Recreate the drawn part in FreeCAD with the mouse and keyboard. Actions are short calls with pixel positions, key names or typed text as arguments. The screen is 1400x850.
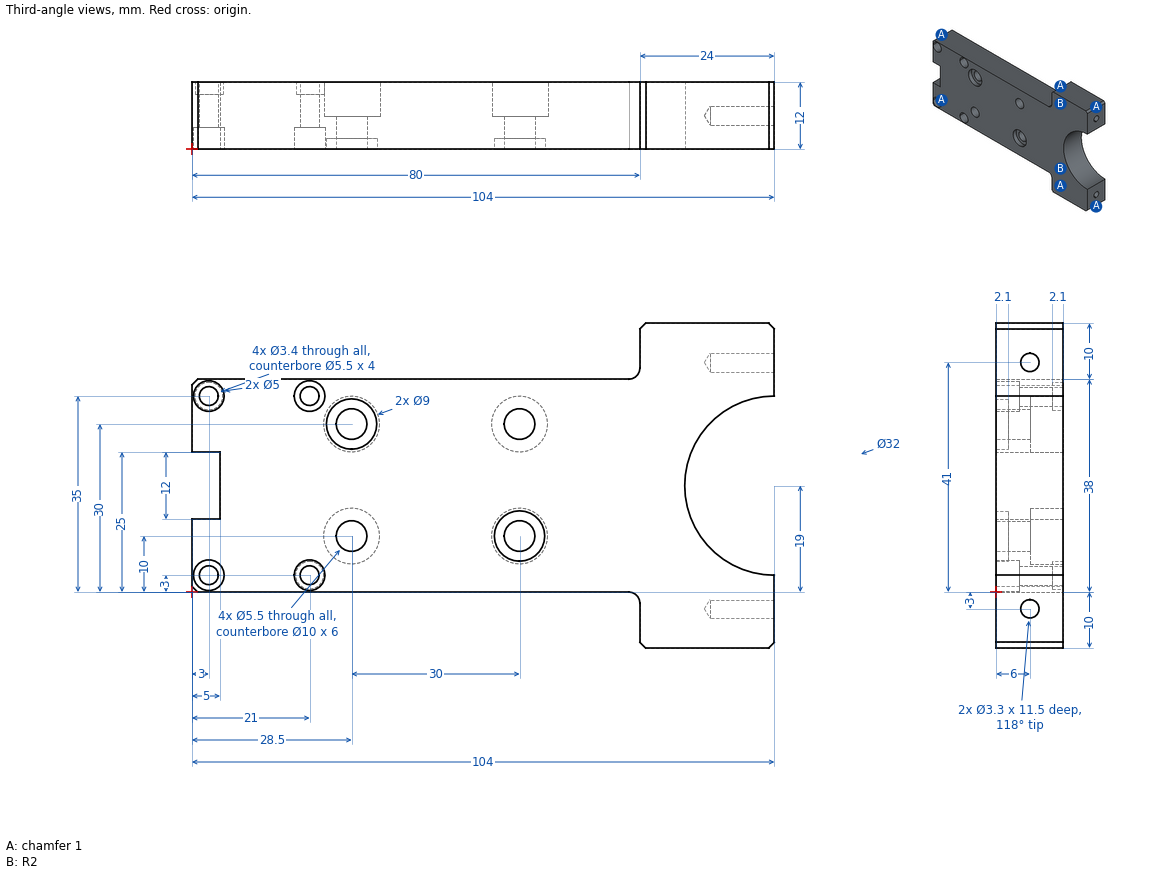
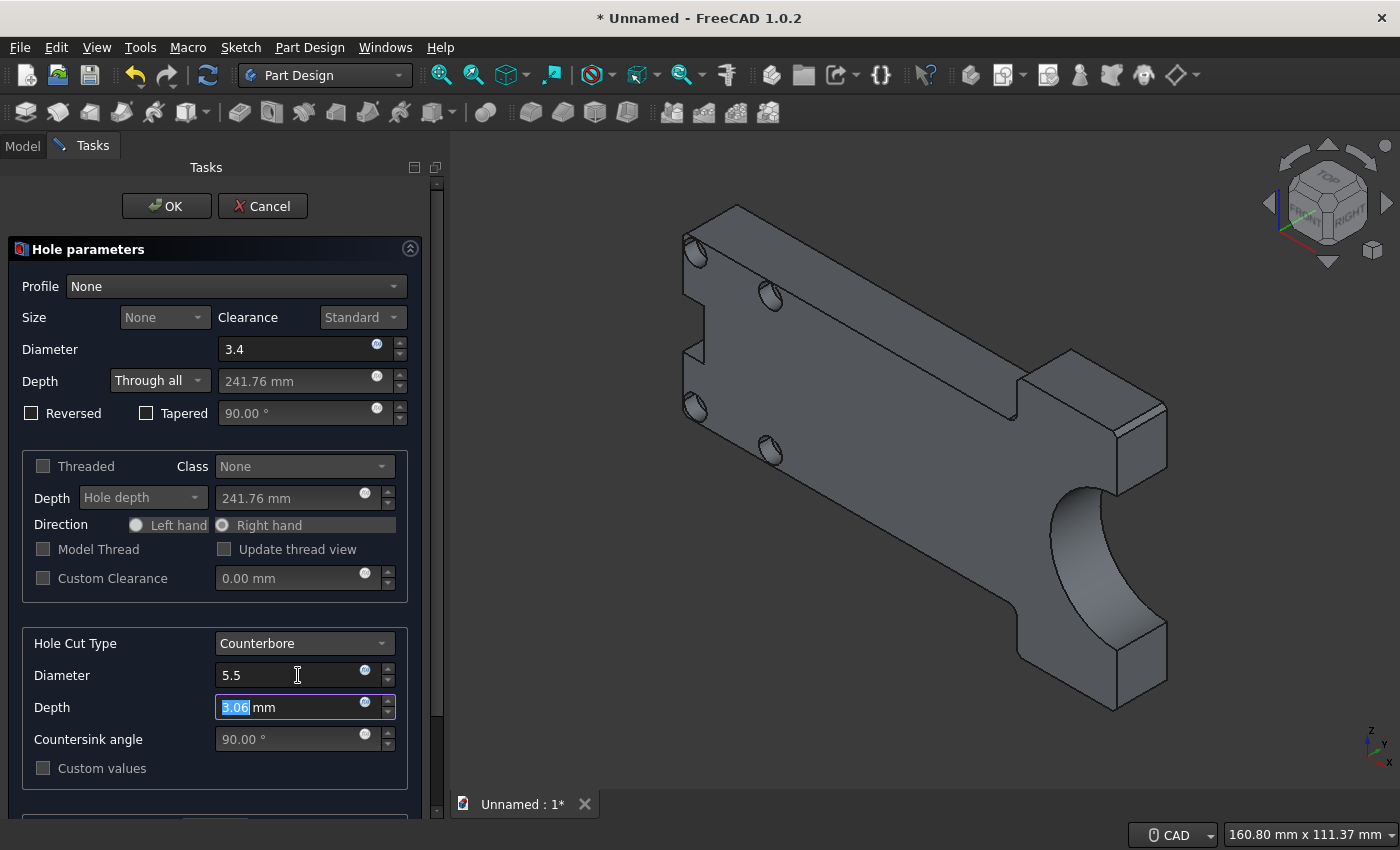
text(4)
key(Tab)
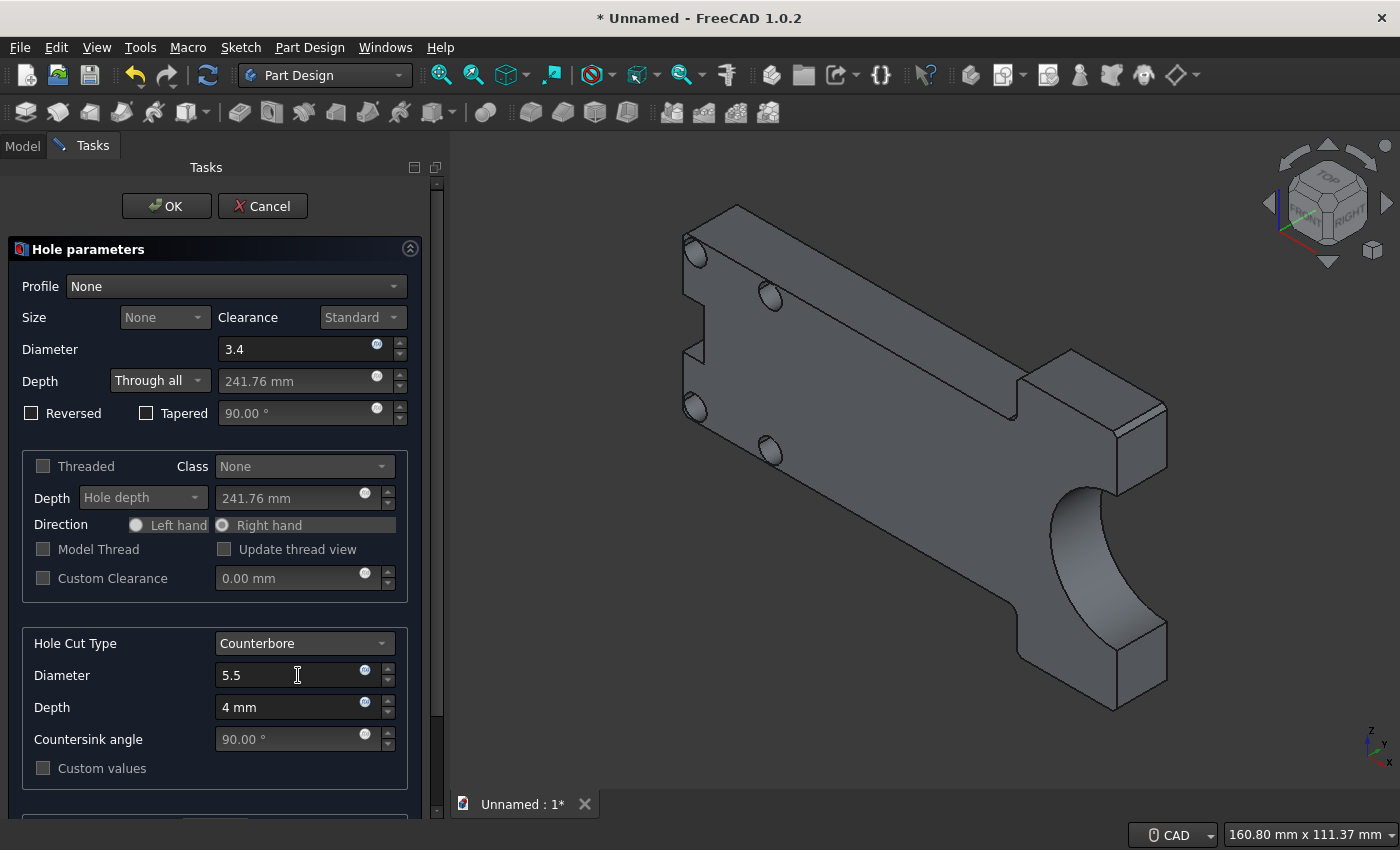
click(167, 206)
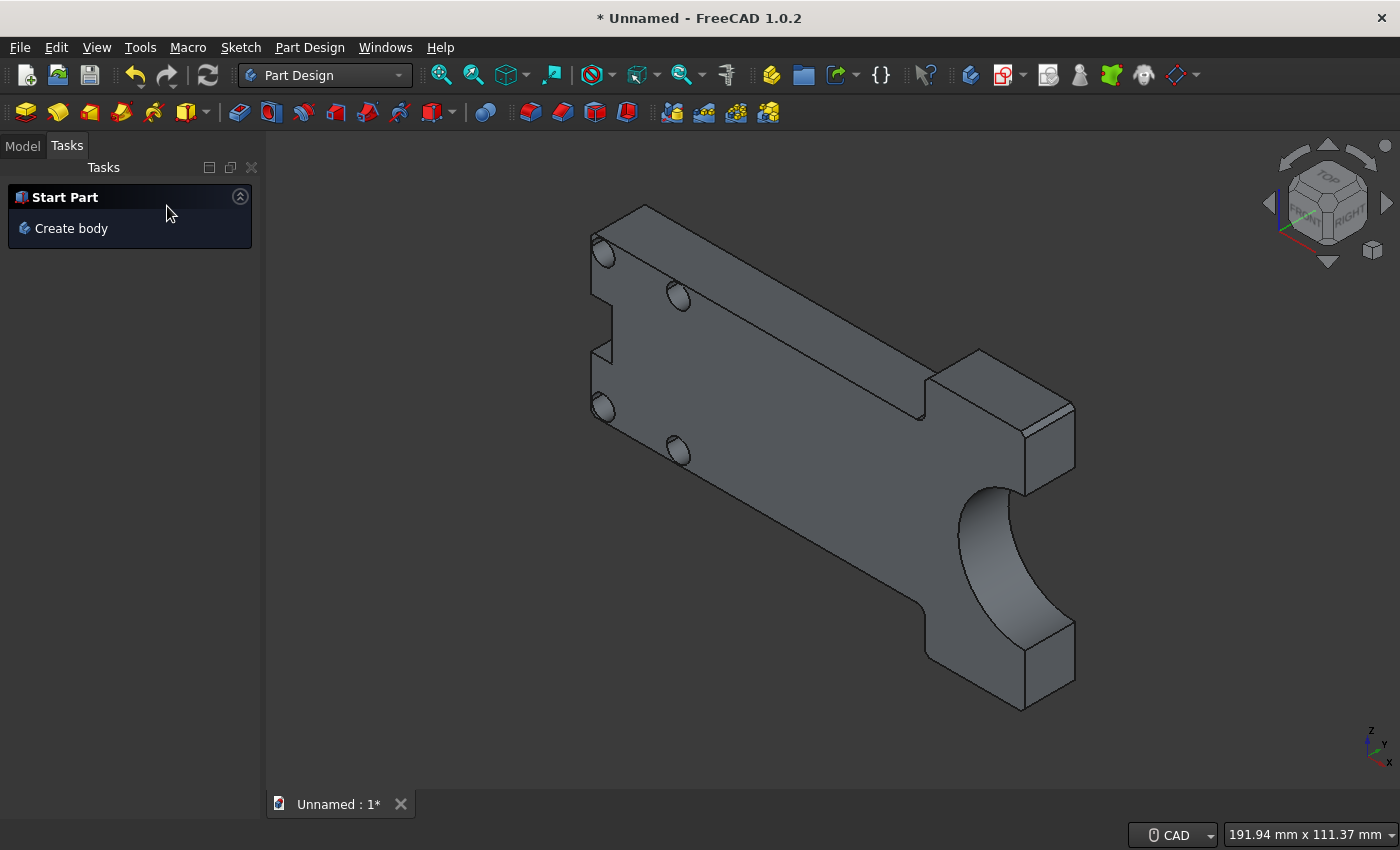
key(4)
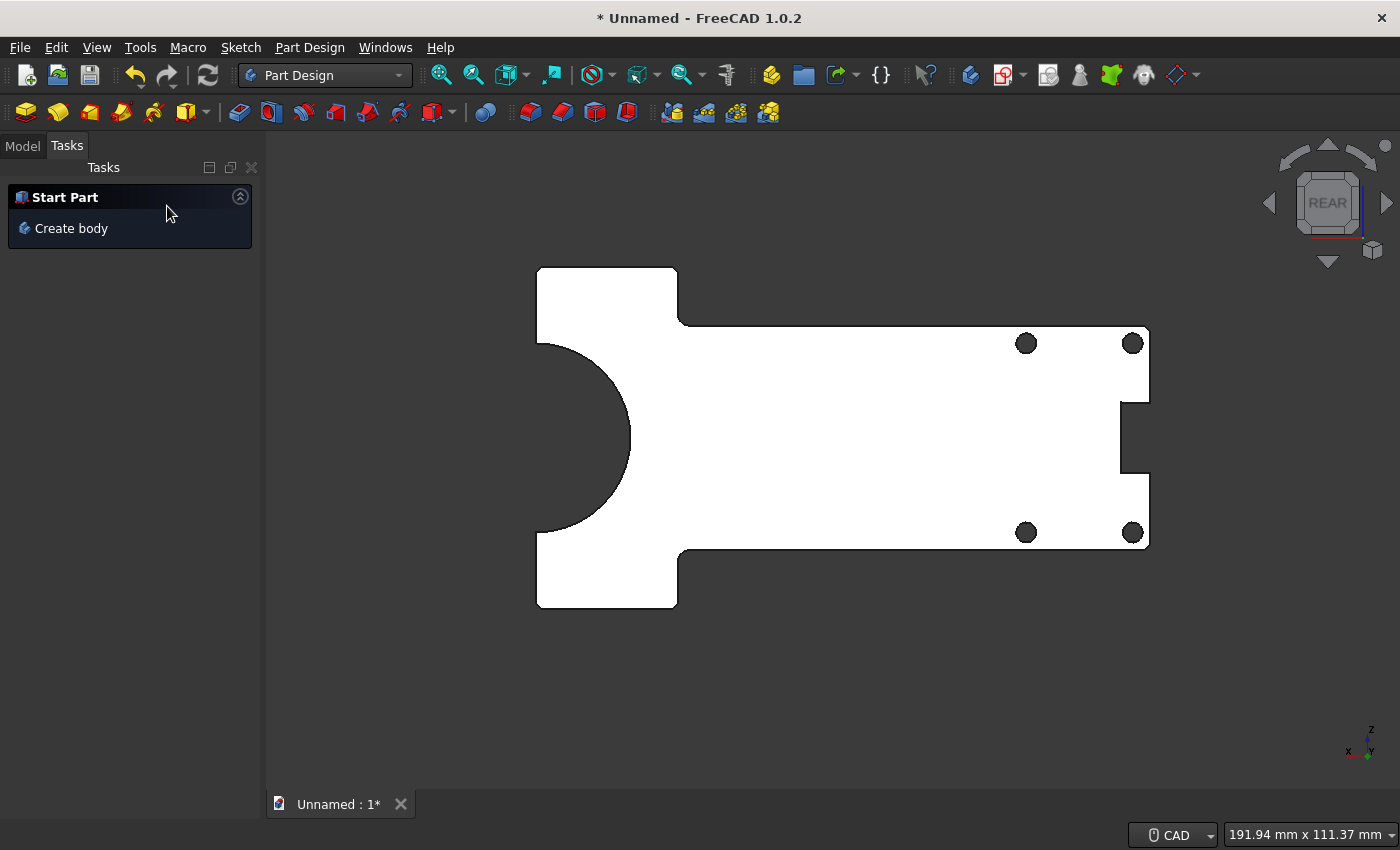
click(755, 437)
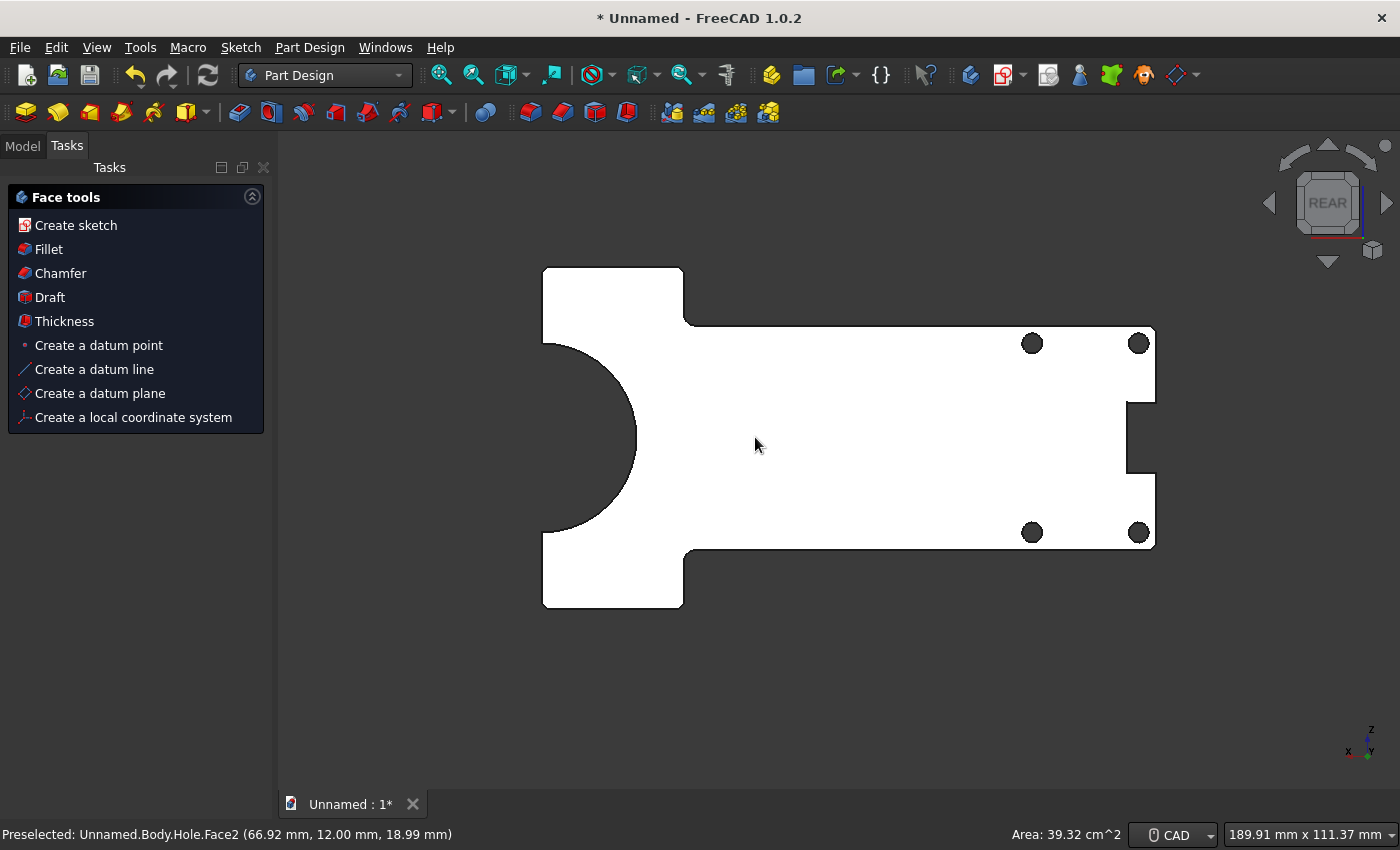
click(1004, 76)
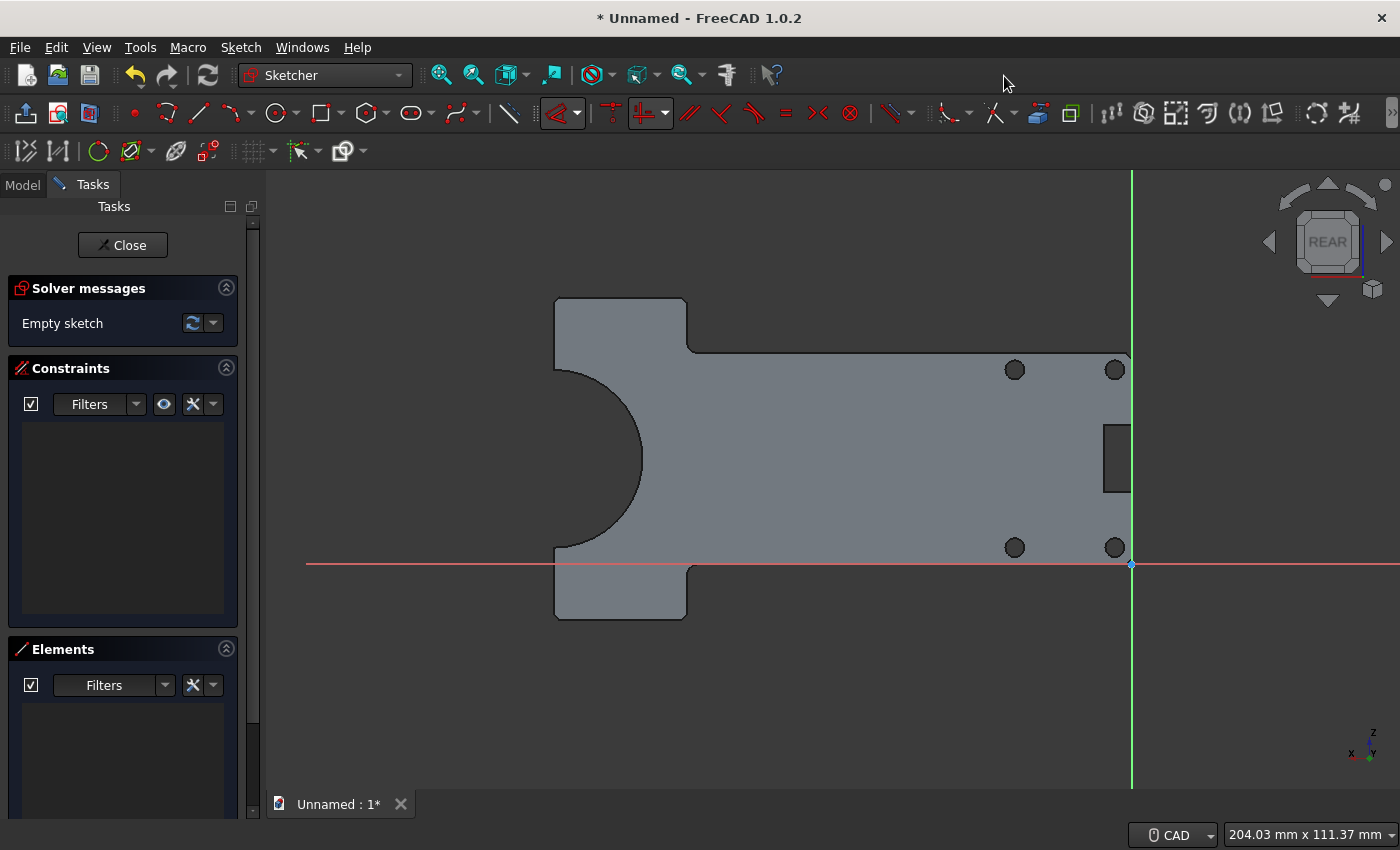
scroll(1235, 437, up, 3)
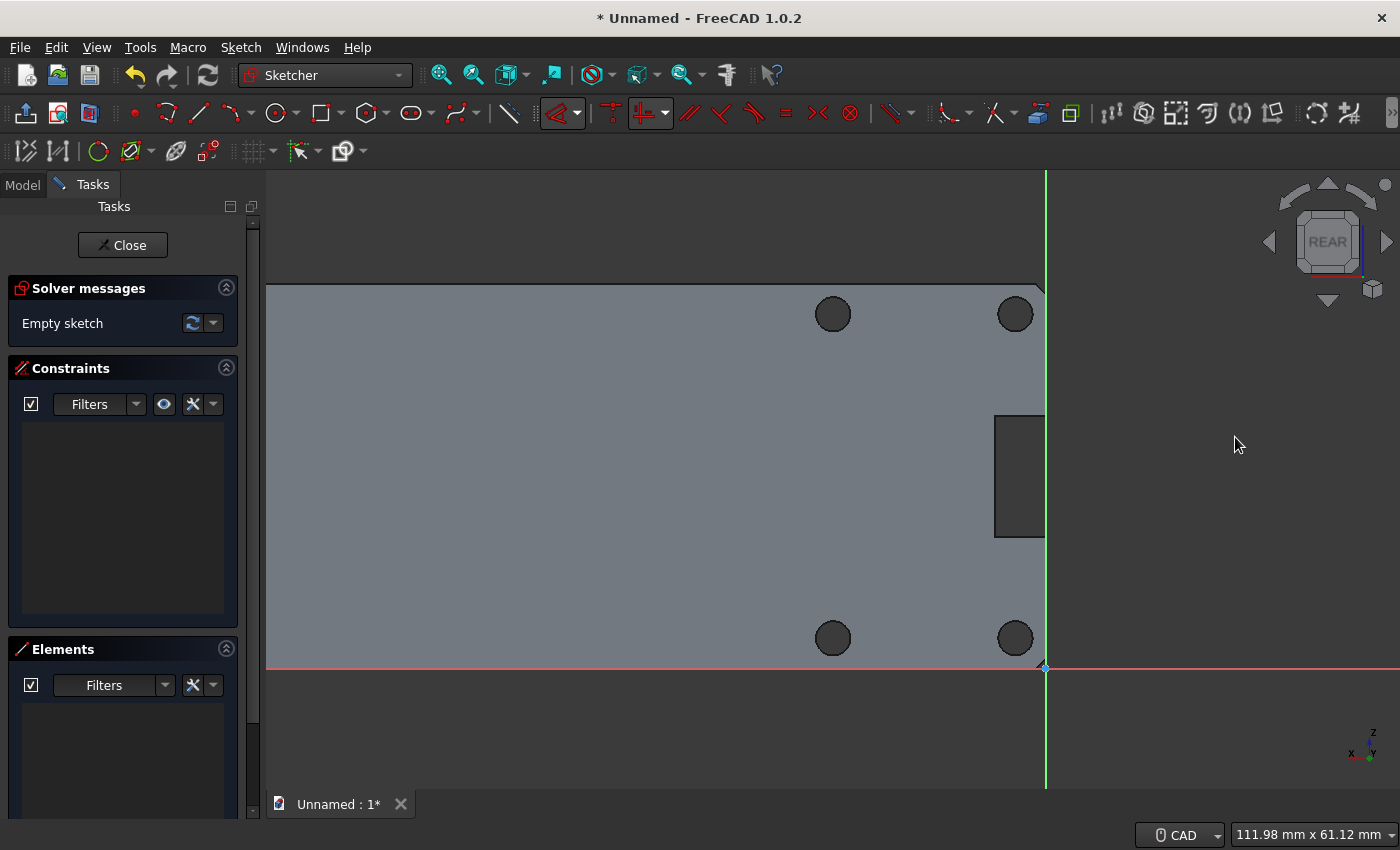
click(276, 114)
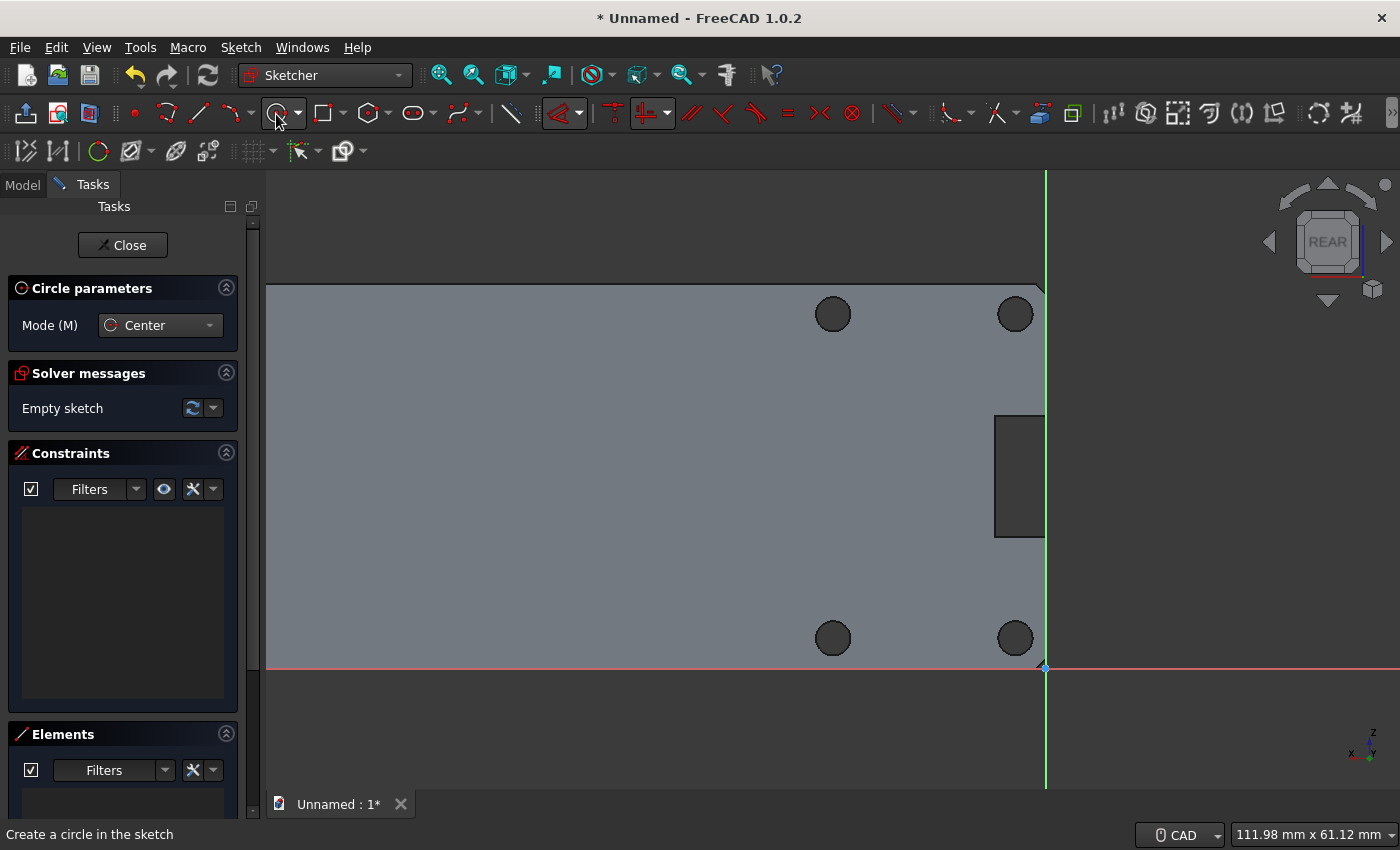
click(1015, 314)
click(998, 296)